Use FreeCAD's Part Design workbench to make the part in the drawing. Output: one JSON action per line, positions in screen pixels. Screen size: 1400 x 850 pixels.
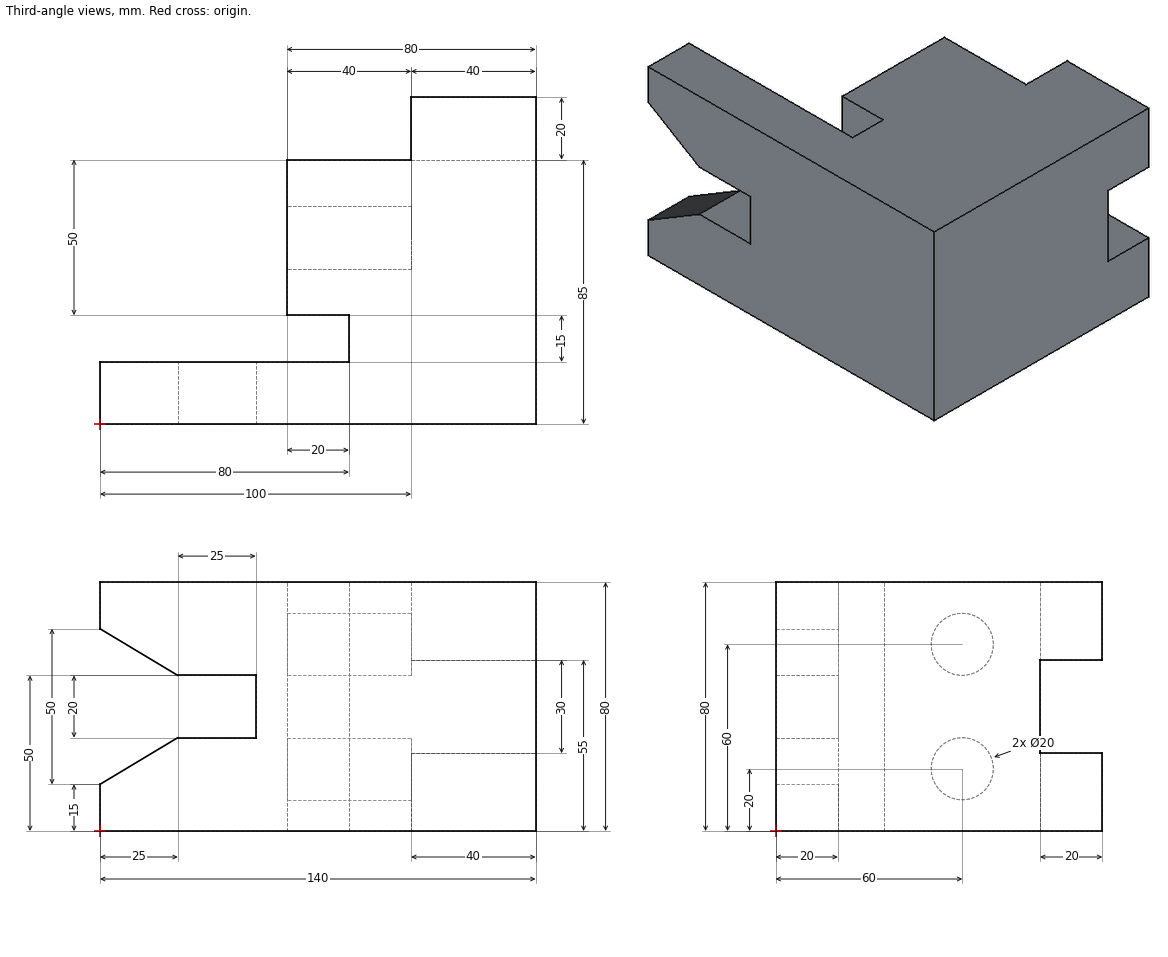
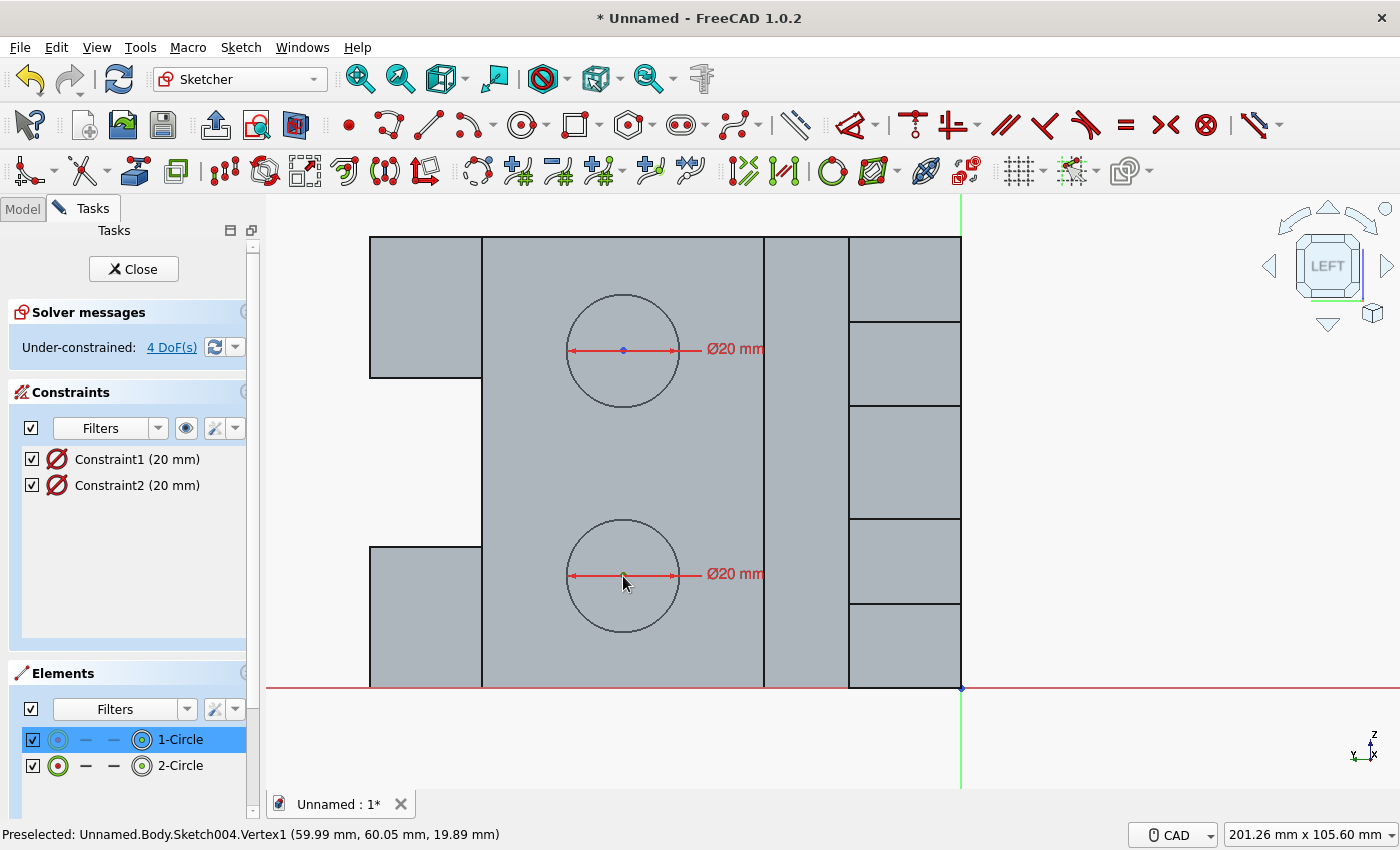
{"action": "left_click", "coordinate": [623, 351]}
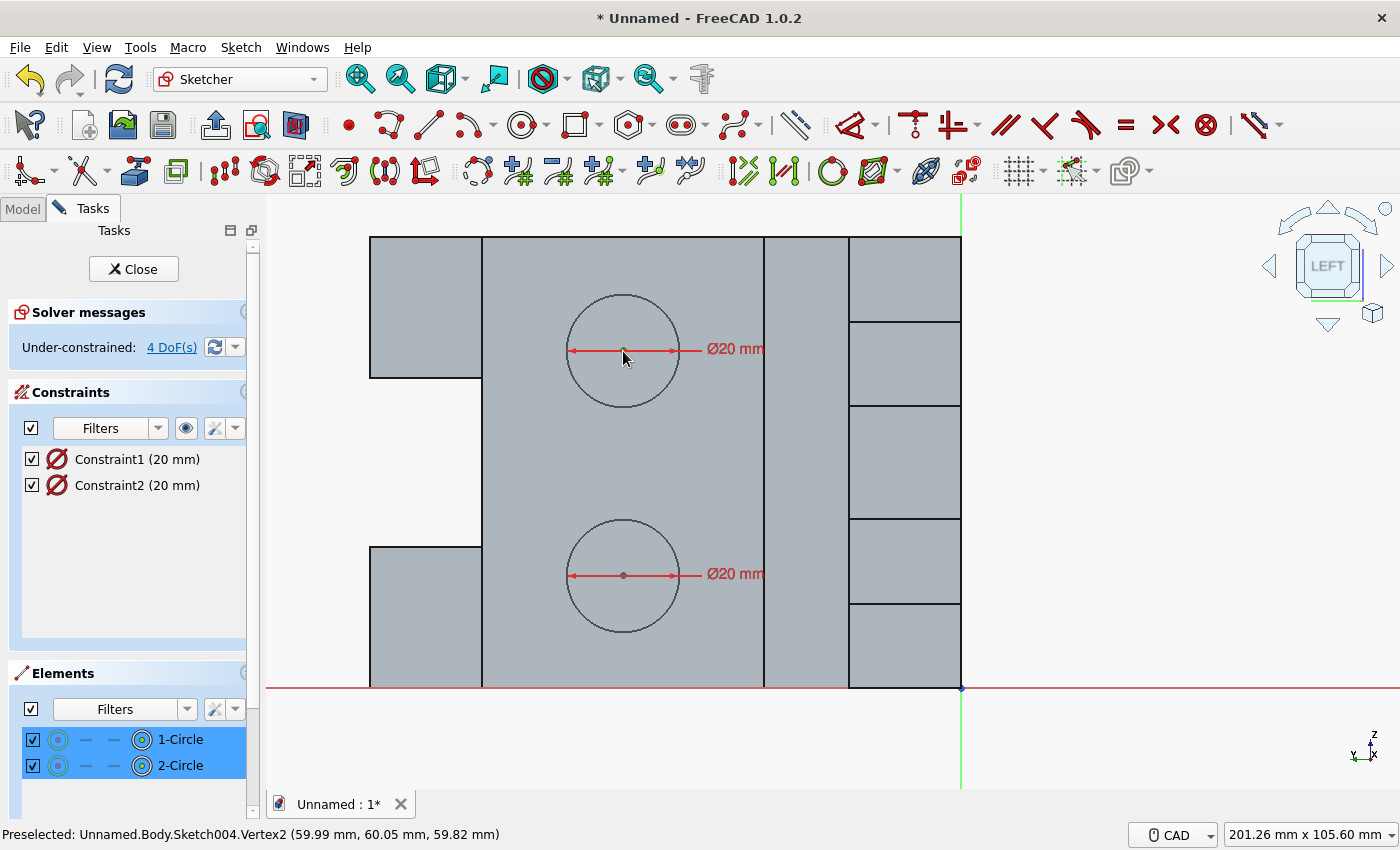
{"action": "left_click", "coordinate": [980, 126]}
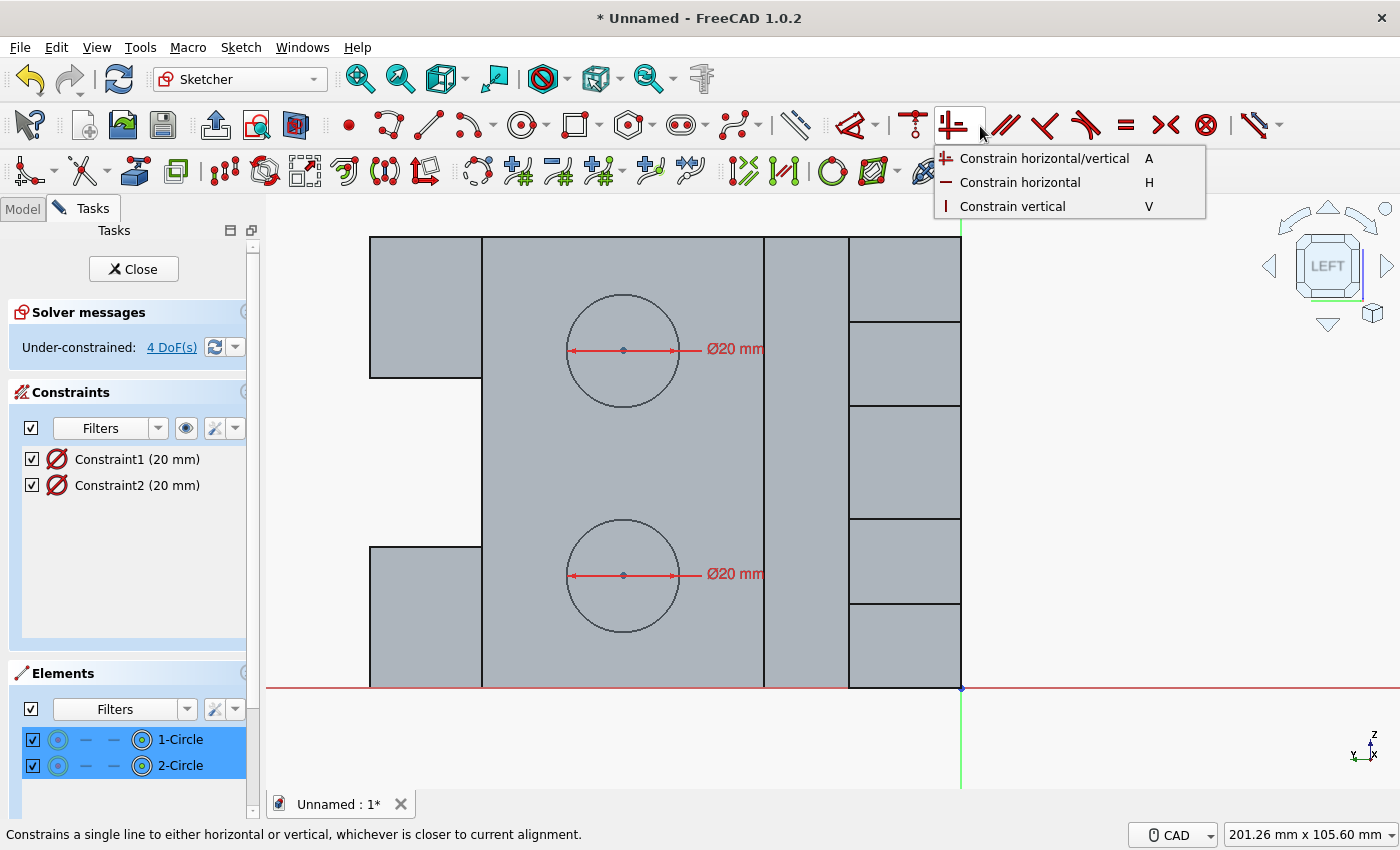
{"action": "left_click", "coordinate": [1070, 206]}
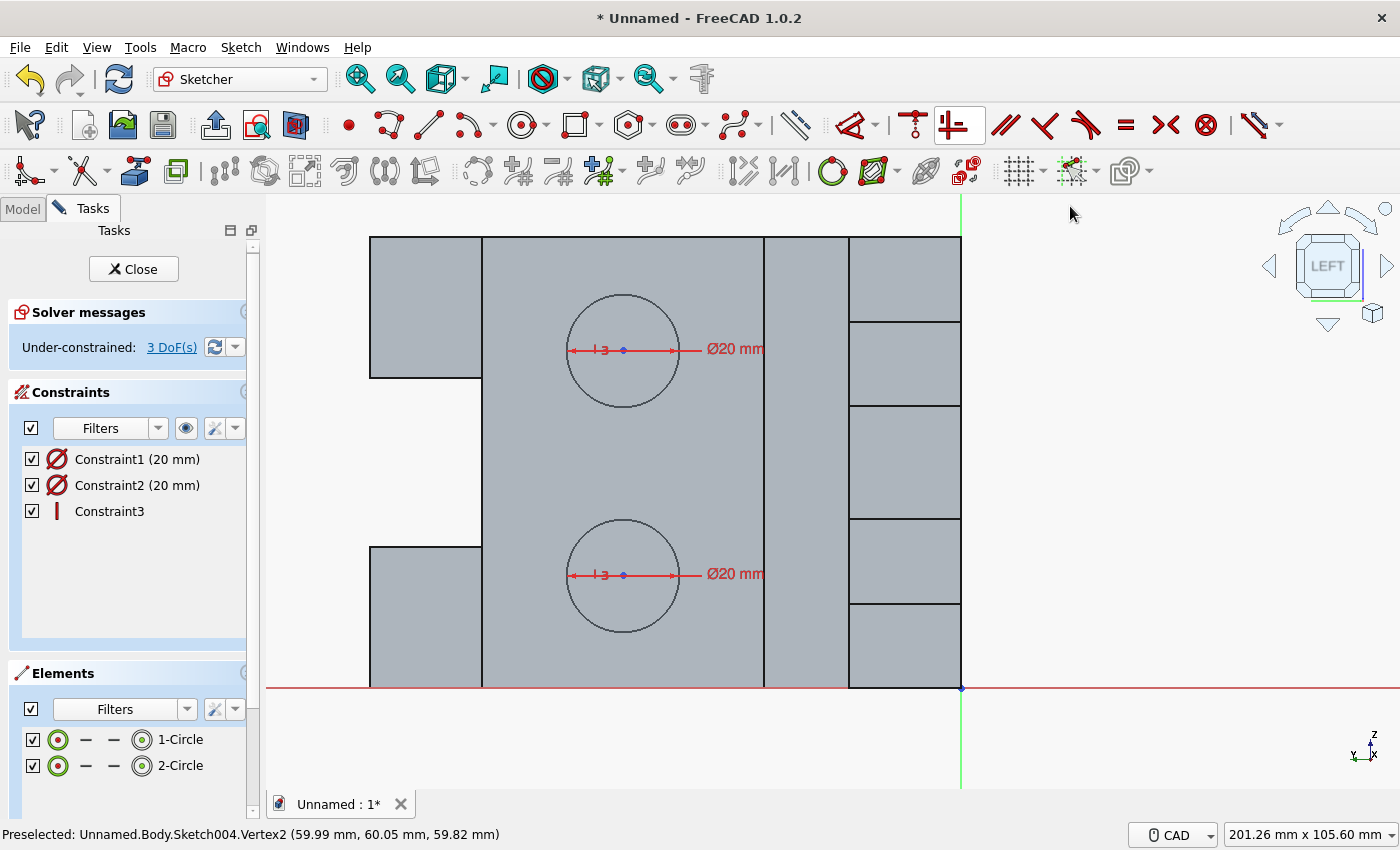
{"action": "left_click", "coordinate": [850, 126]}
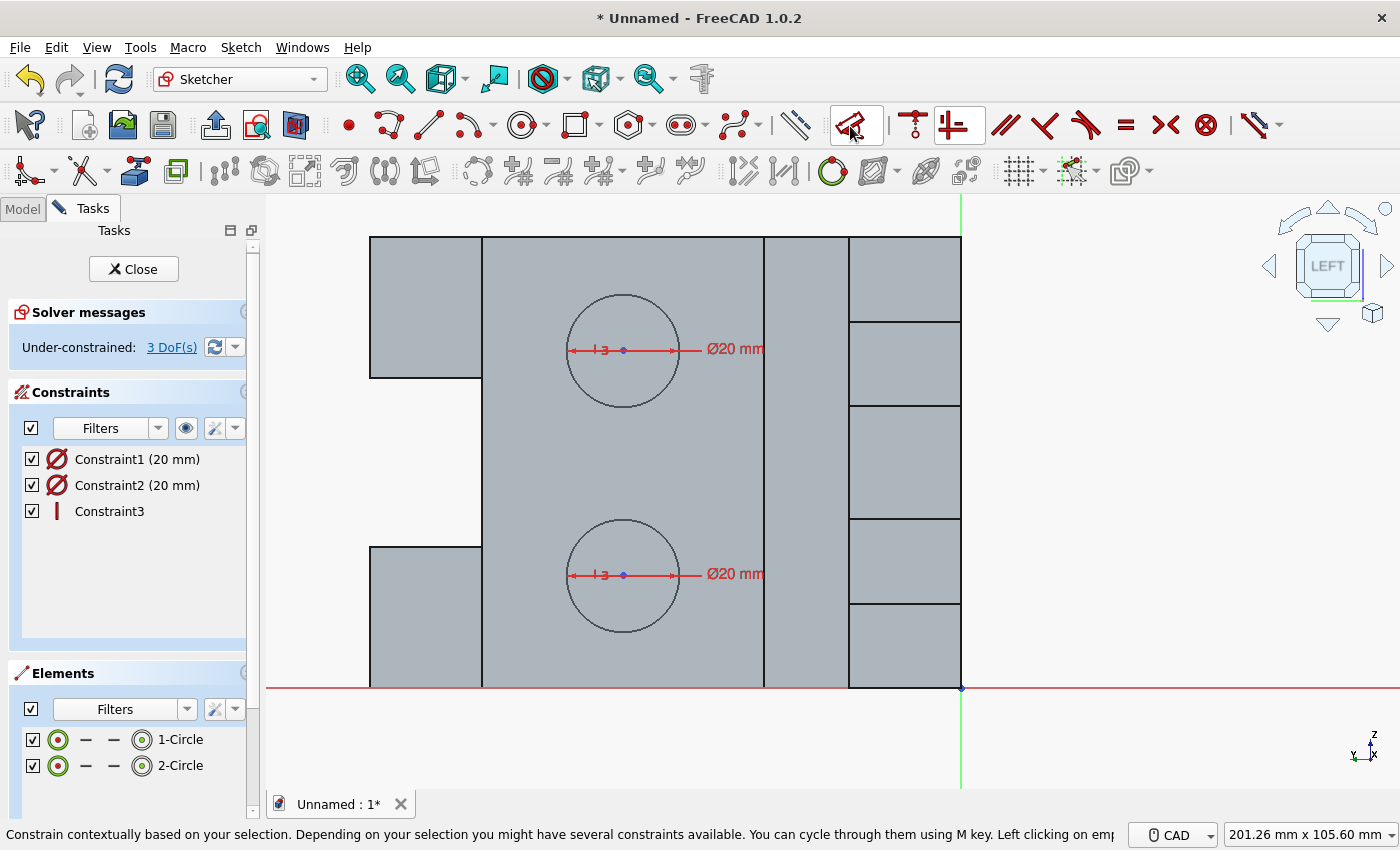
{"action": "left_click", "coordinate": [623, 576]}
{"action": "left_click", "coordinate": [792, 722]}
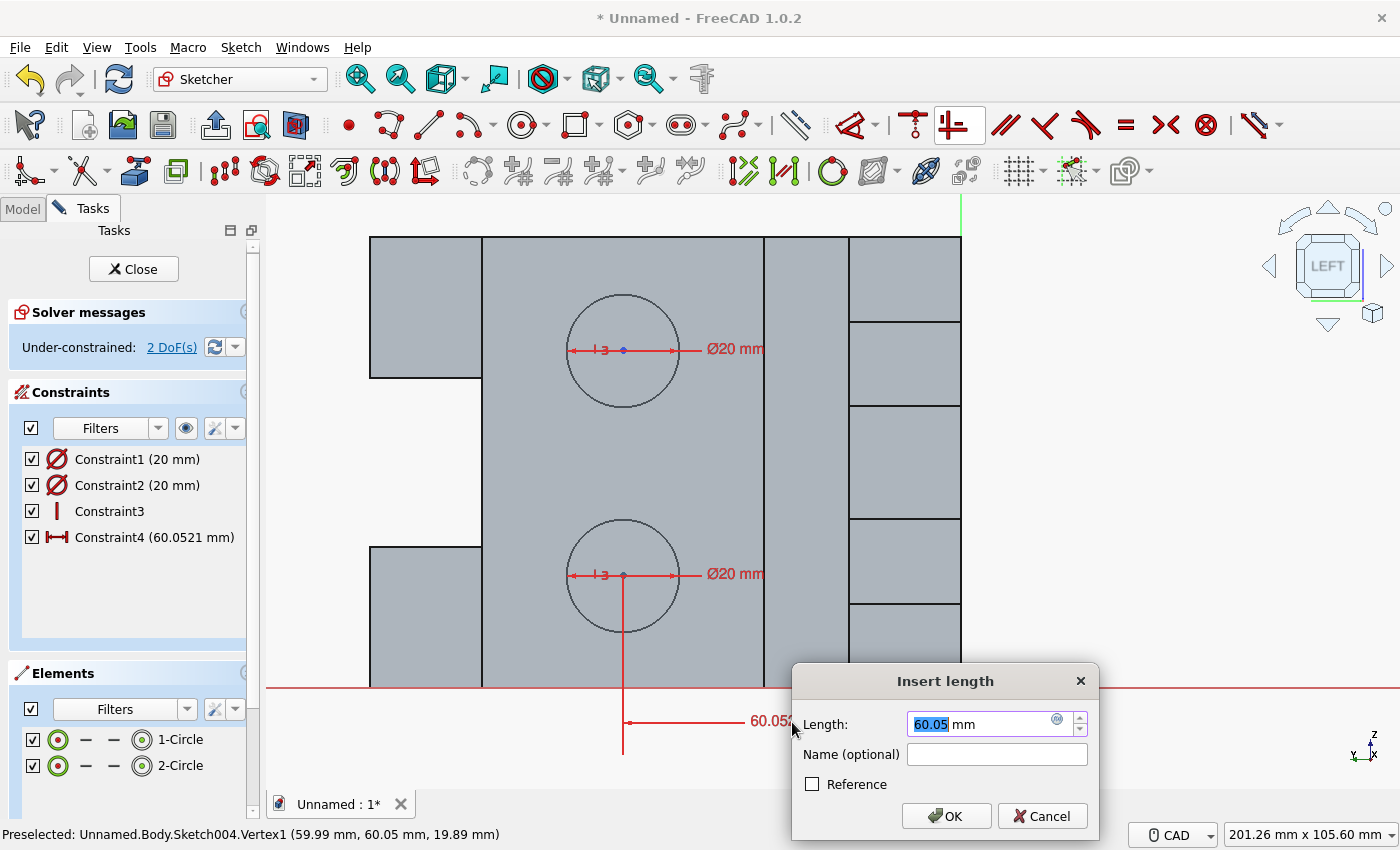
{"action": "type", "text": "60"}
{"action": "key", "text": "Return"}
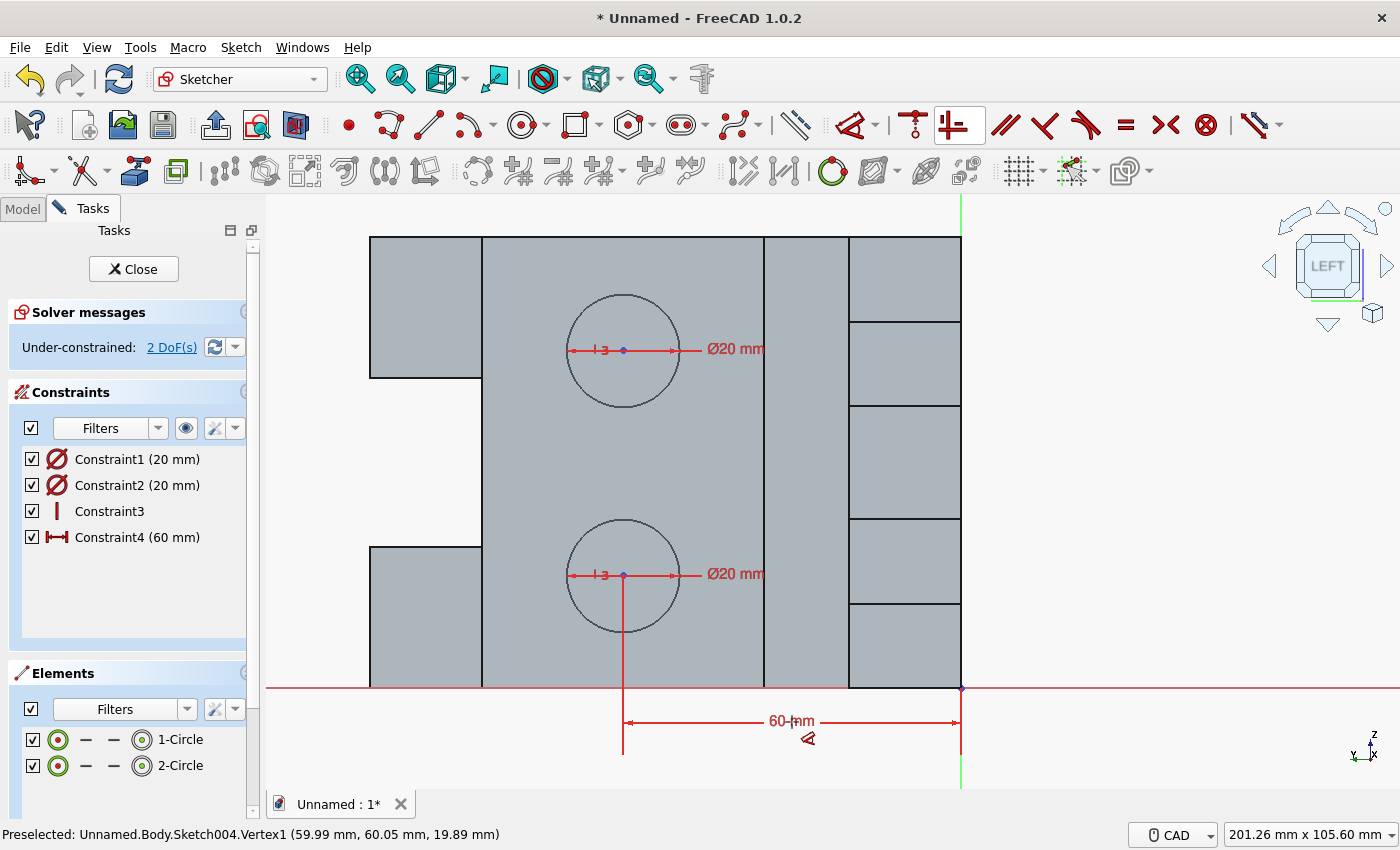
{"action": "left_click", "coordinate": [623, 576]}
{"action": "left_click", "coordinate": [995, 632]}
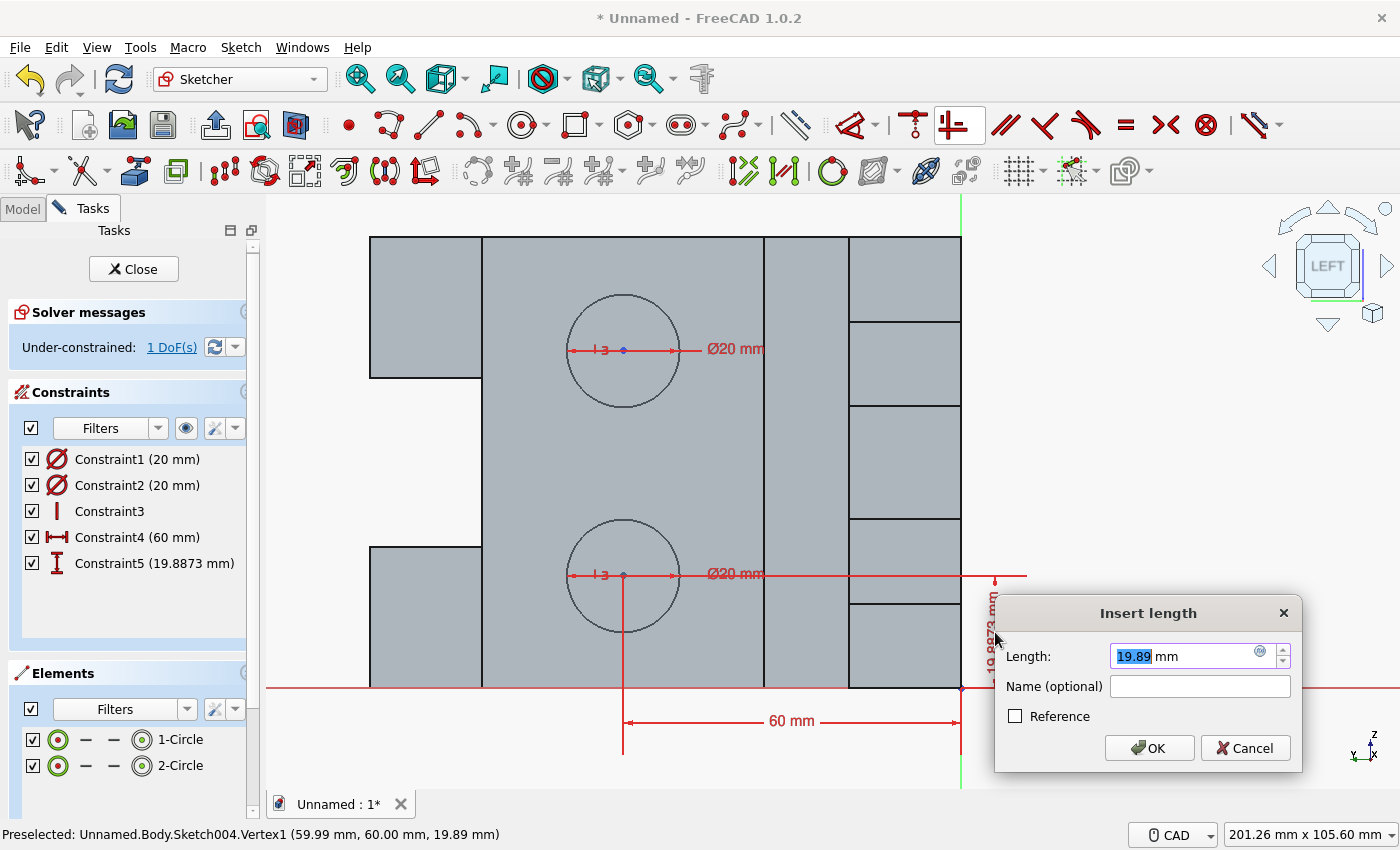
{"action": "type", "text": "20"}
{"action": "key", "text": "Return"}